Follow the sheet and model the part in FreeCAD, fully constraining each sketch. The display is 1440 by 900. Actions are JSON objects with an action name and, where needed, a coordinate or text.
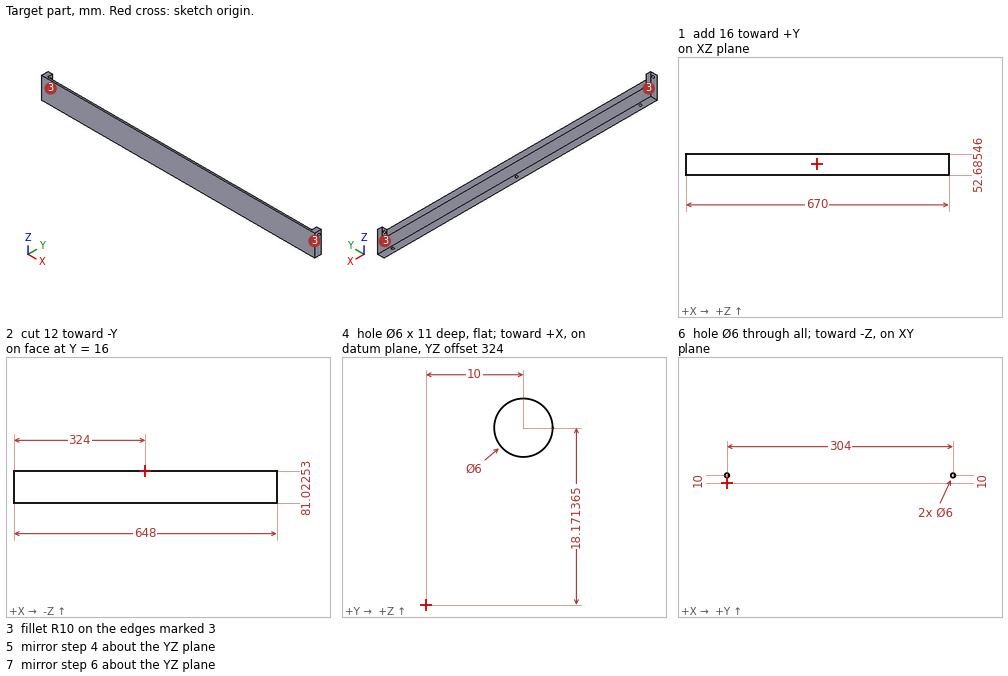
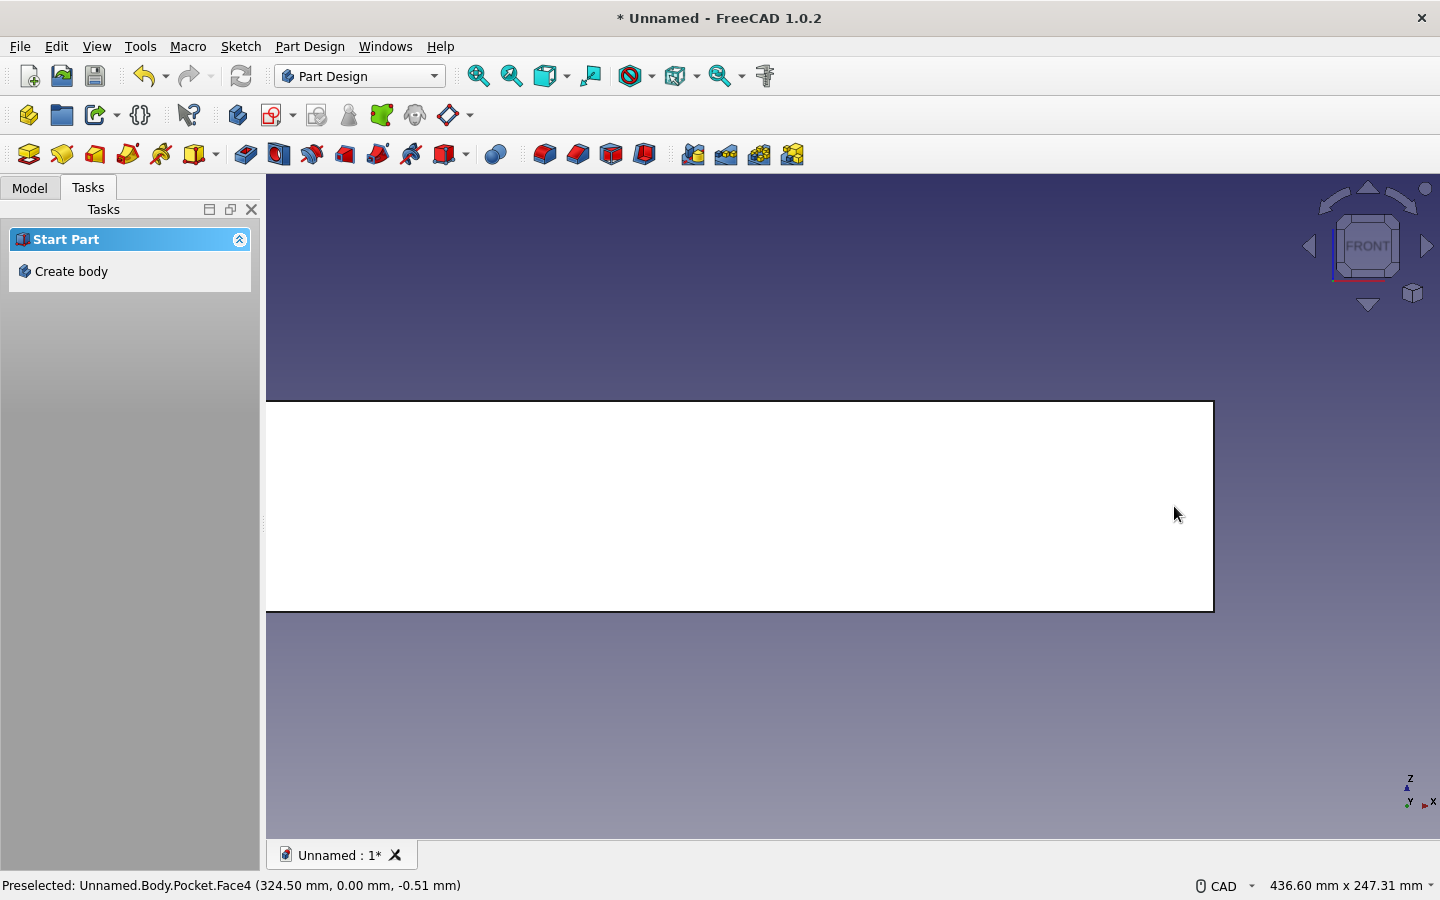
{"action": "left_click", "coordinate": [479, 76]}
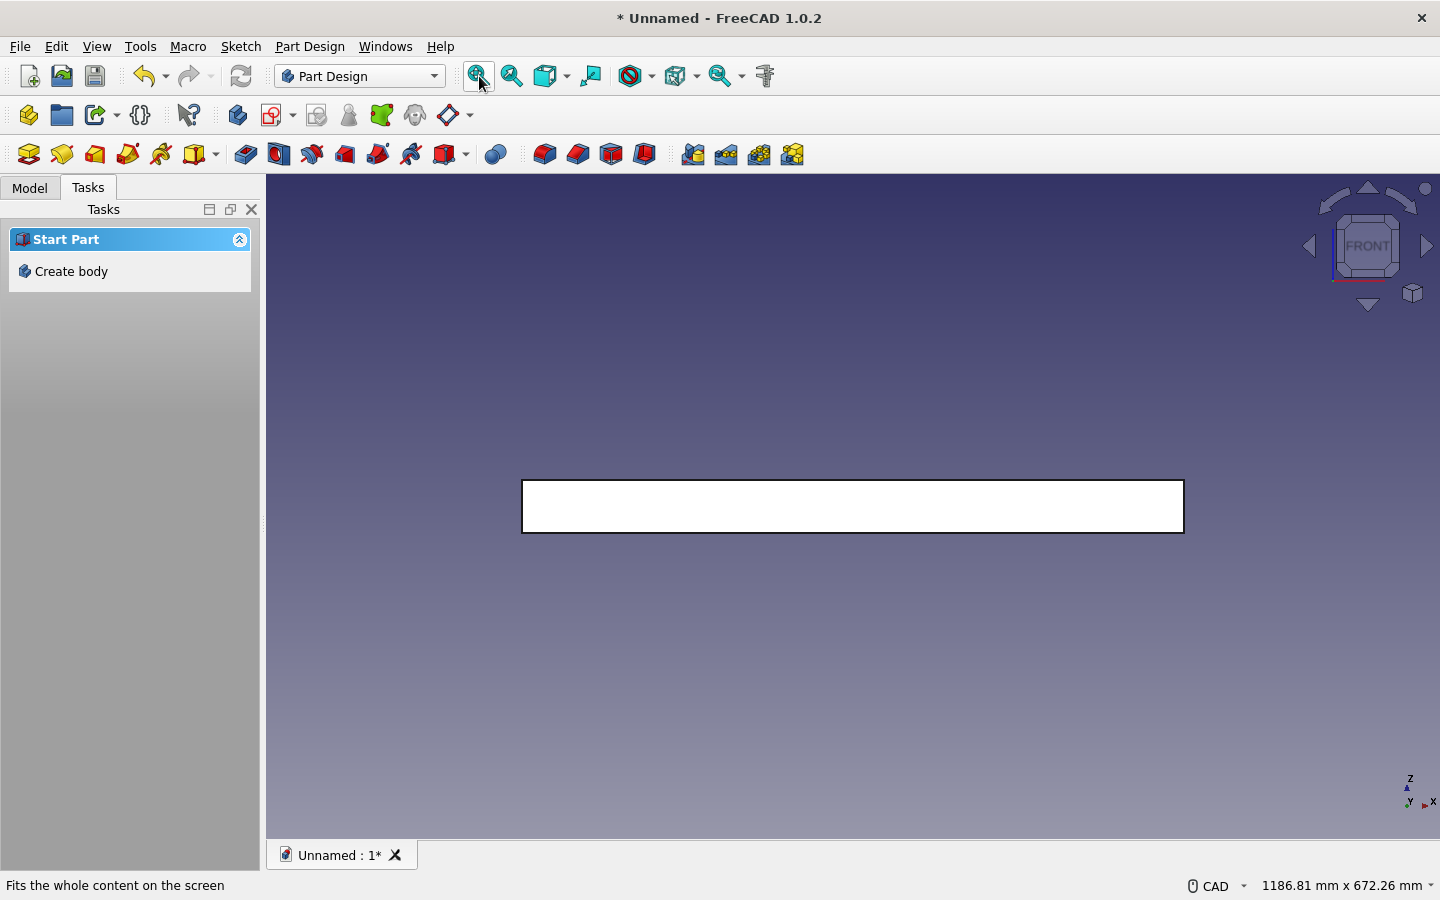
{"action": "key", "text": "3"}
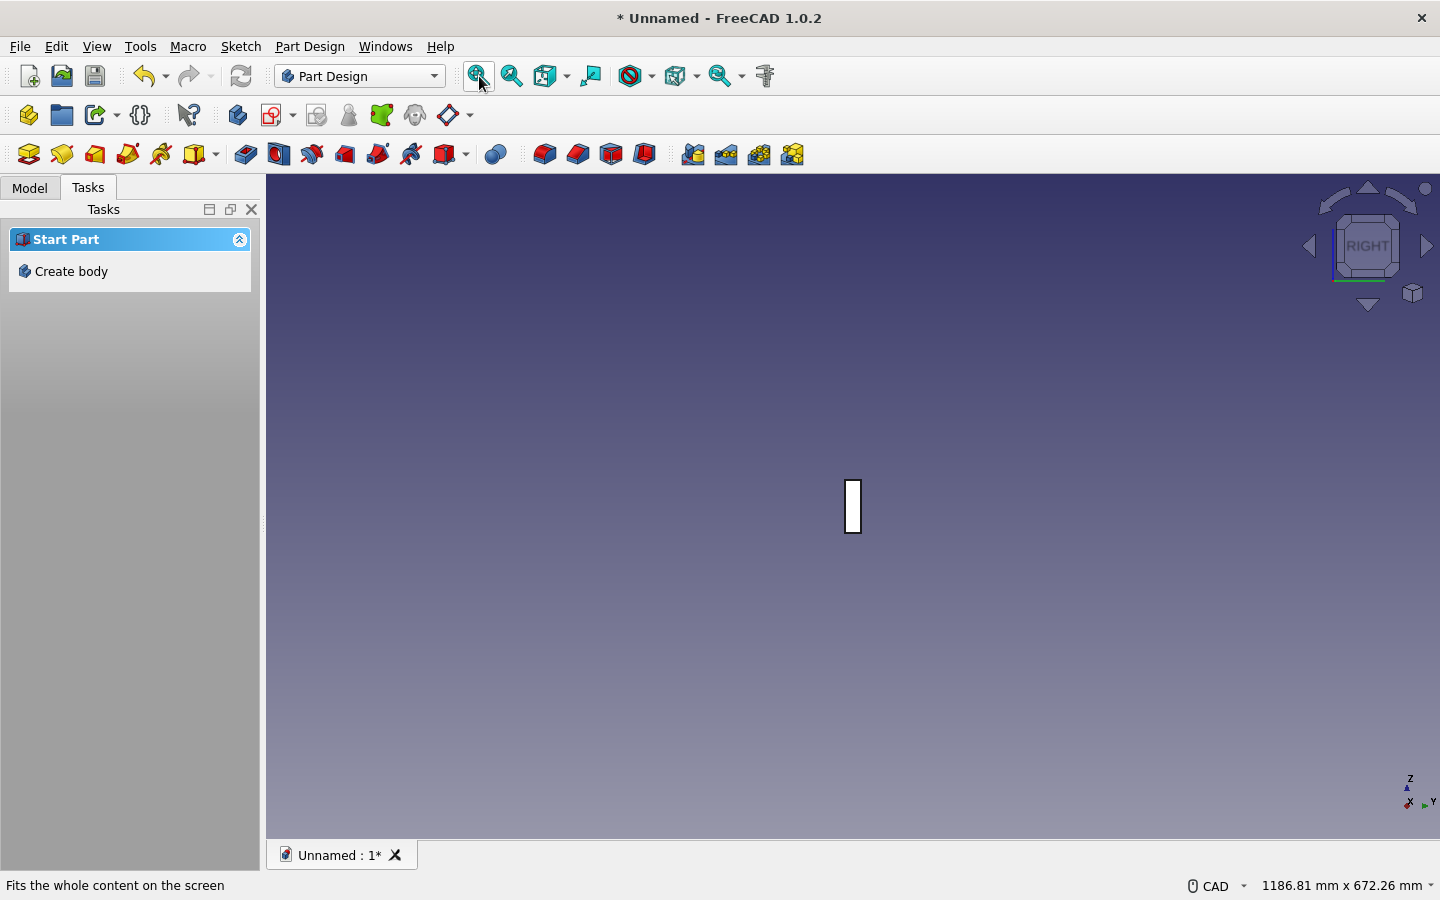
{"action": "left_click", "coordinate": [479, 76]}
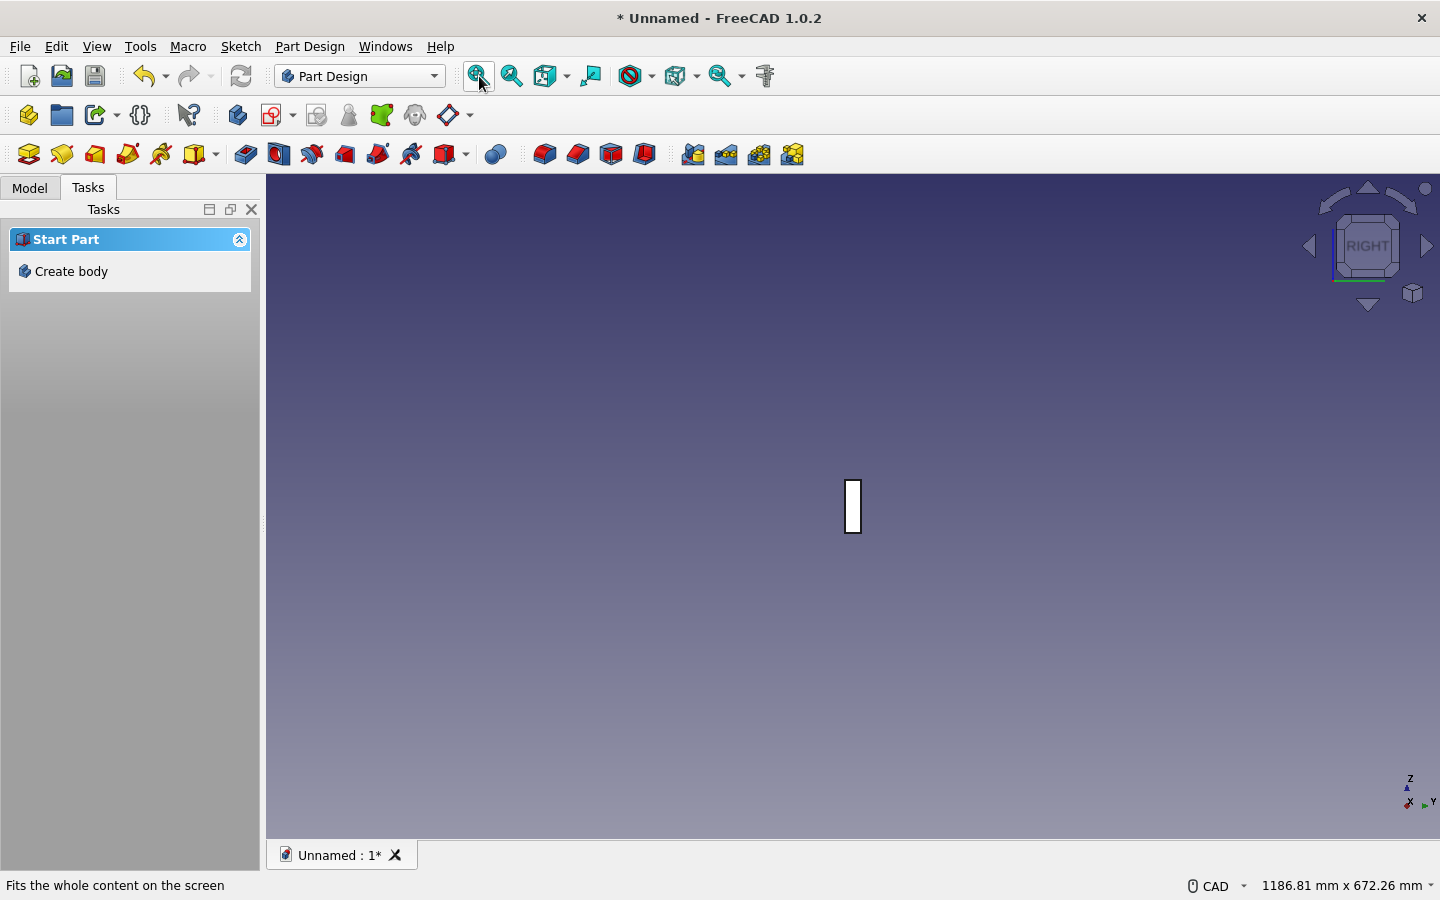
{"action": "scroll", "coordinate": [855, 505], "scroll_direction": "up", "scroll_amount": 7}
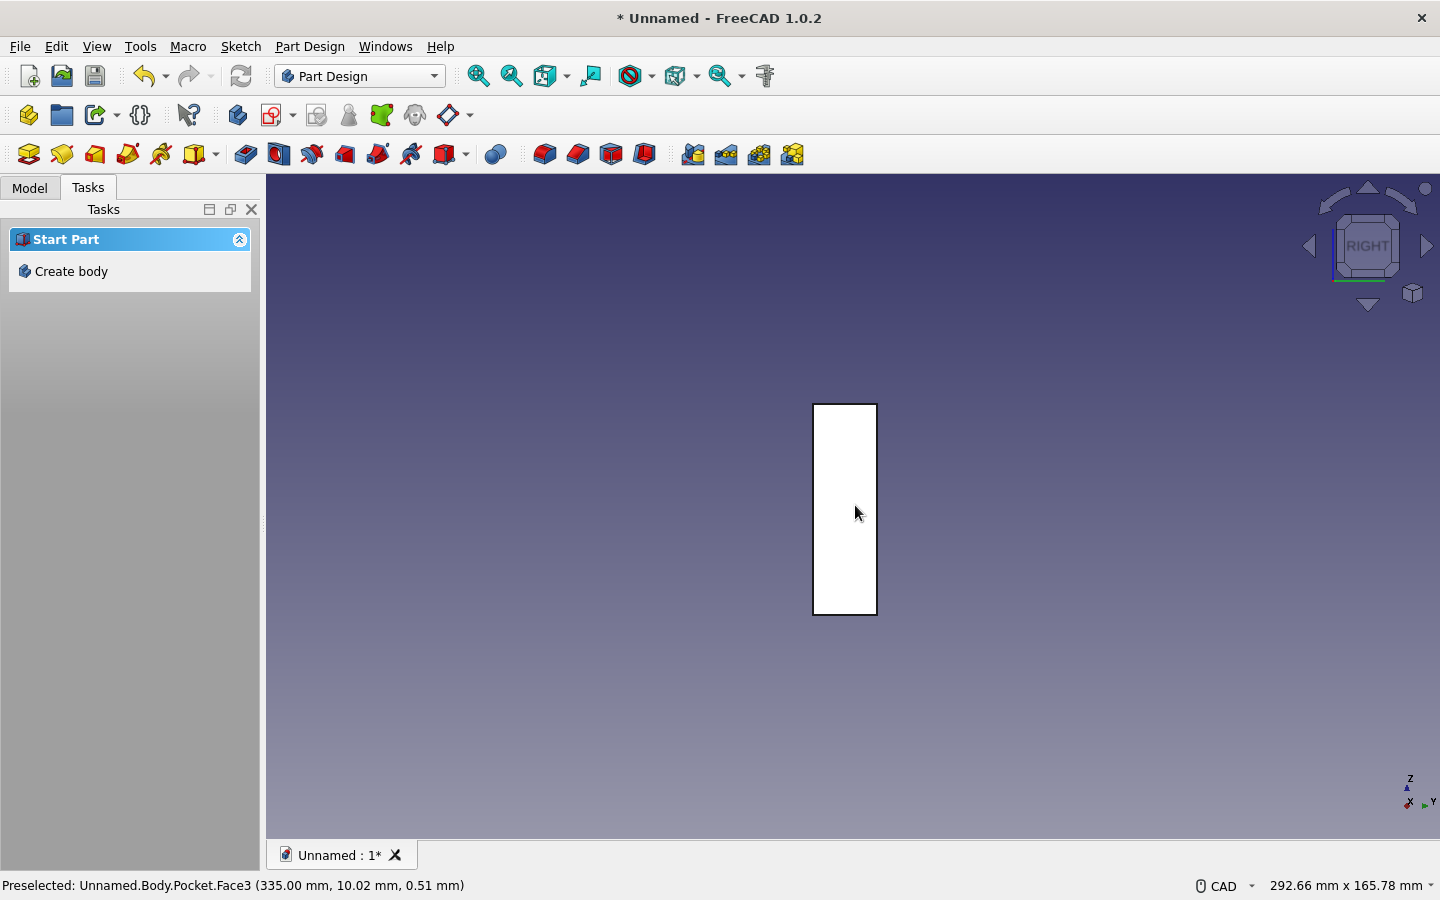
{"action": "left_click", "coordinate": [479, 76]}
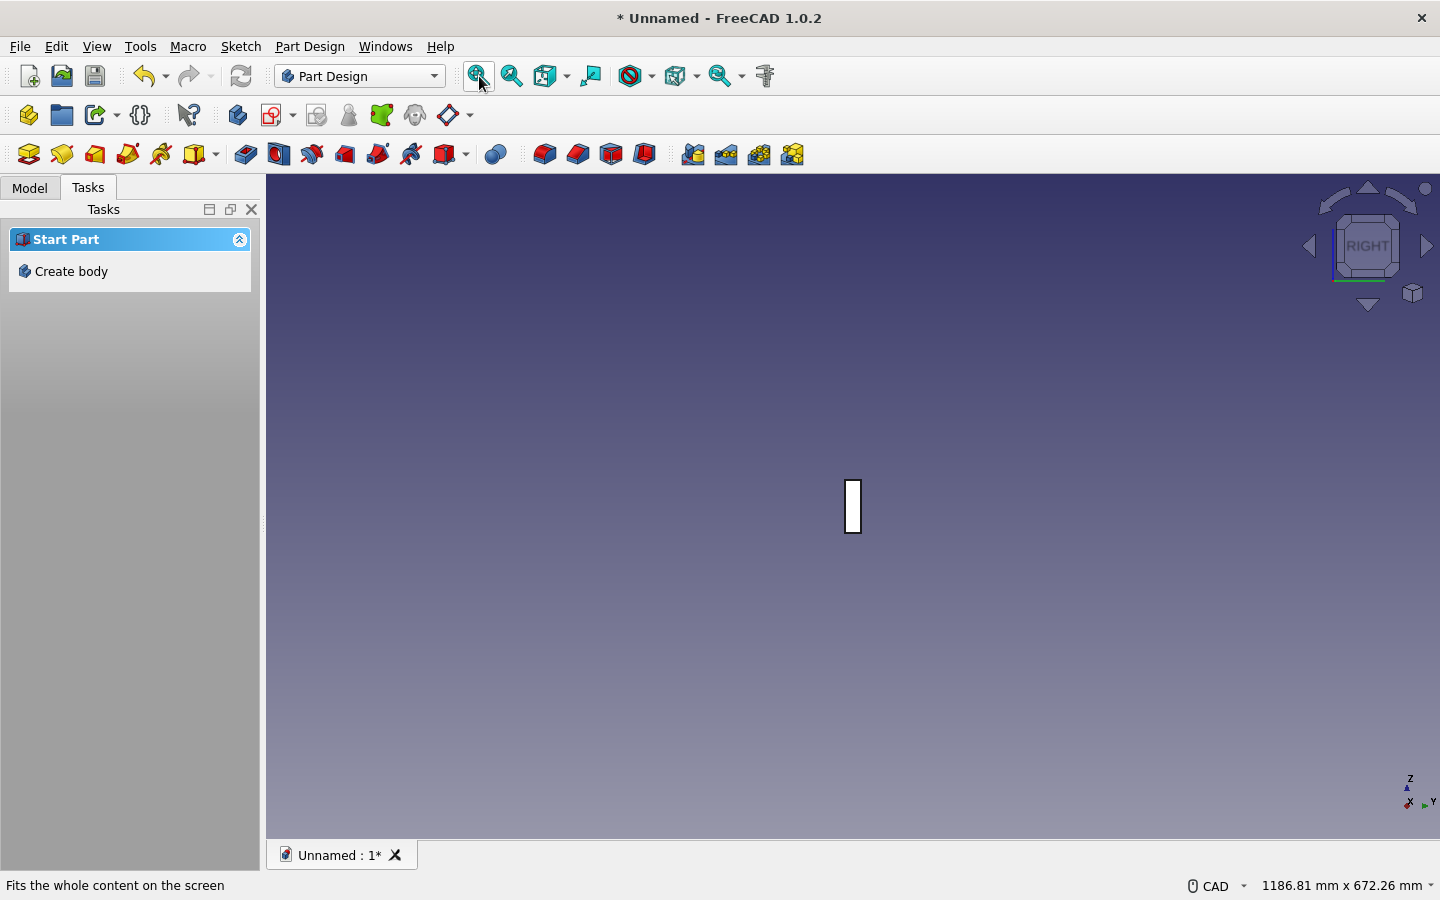
{"action": "key", "text": "5"}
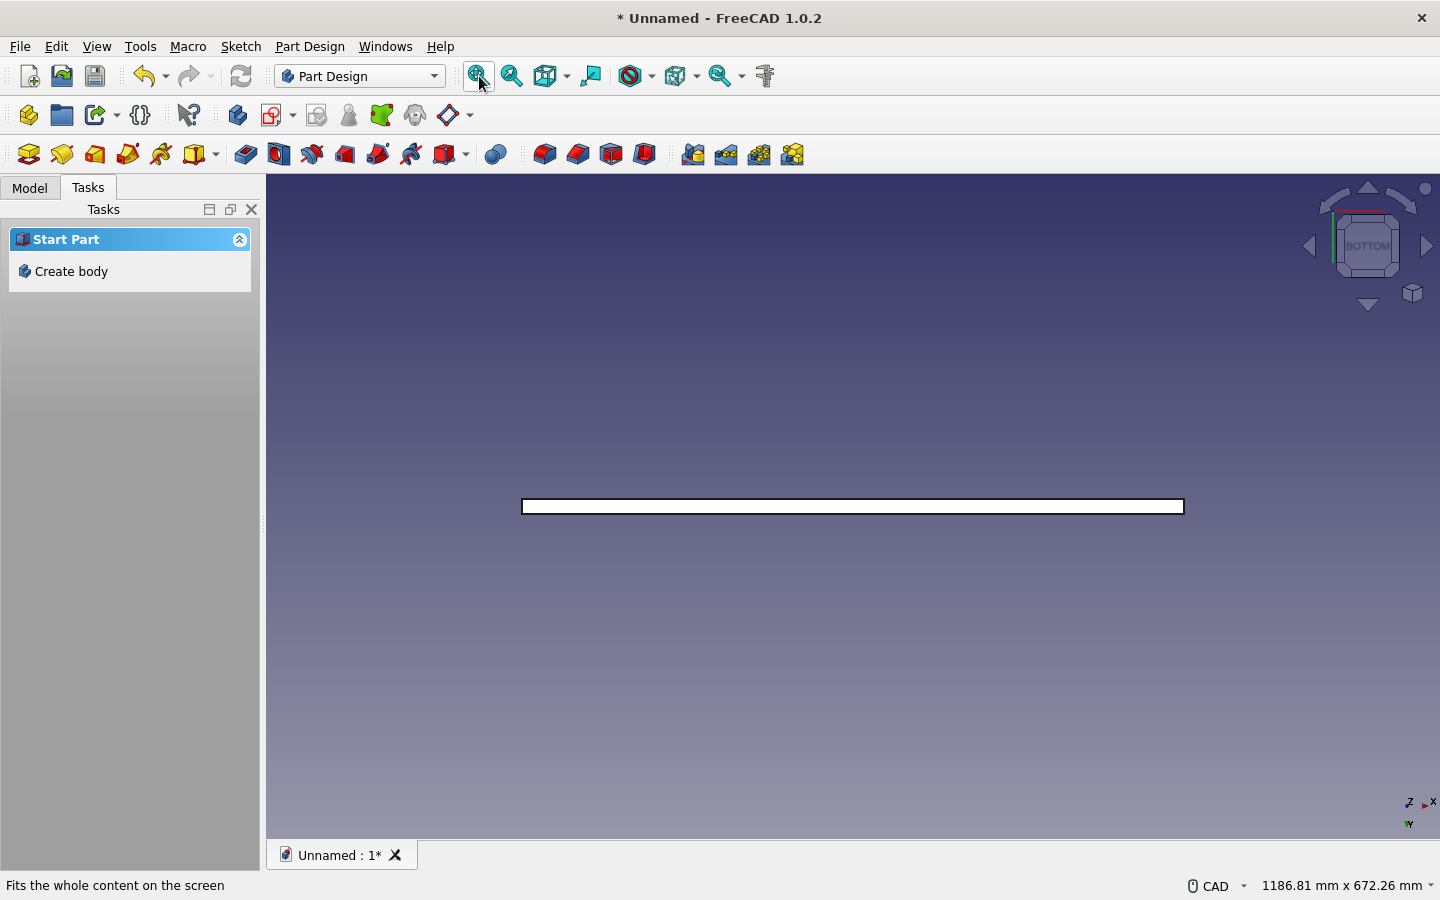
{"action": "scroll", "coordinate": [1174, 507], "scroll_direction": "up", "scroll_amount": 7}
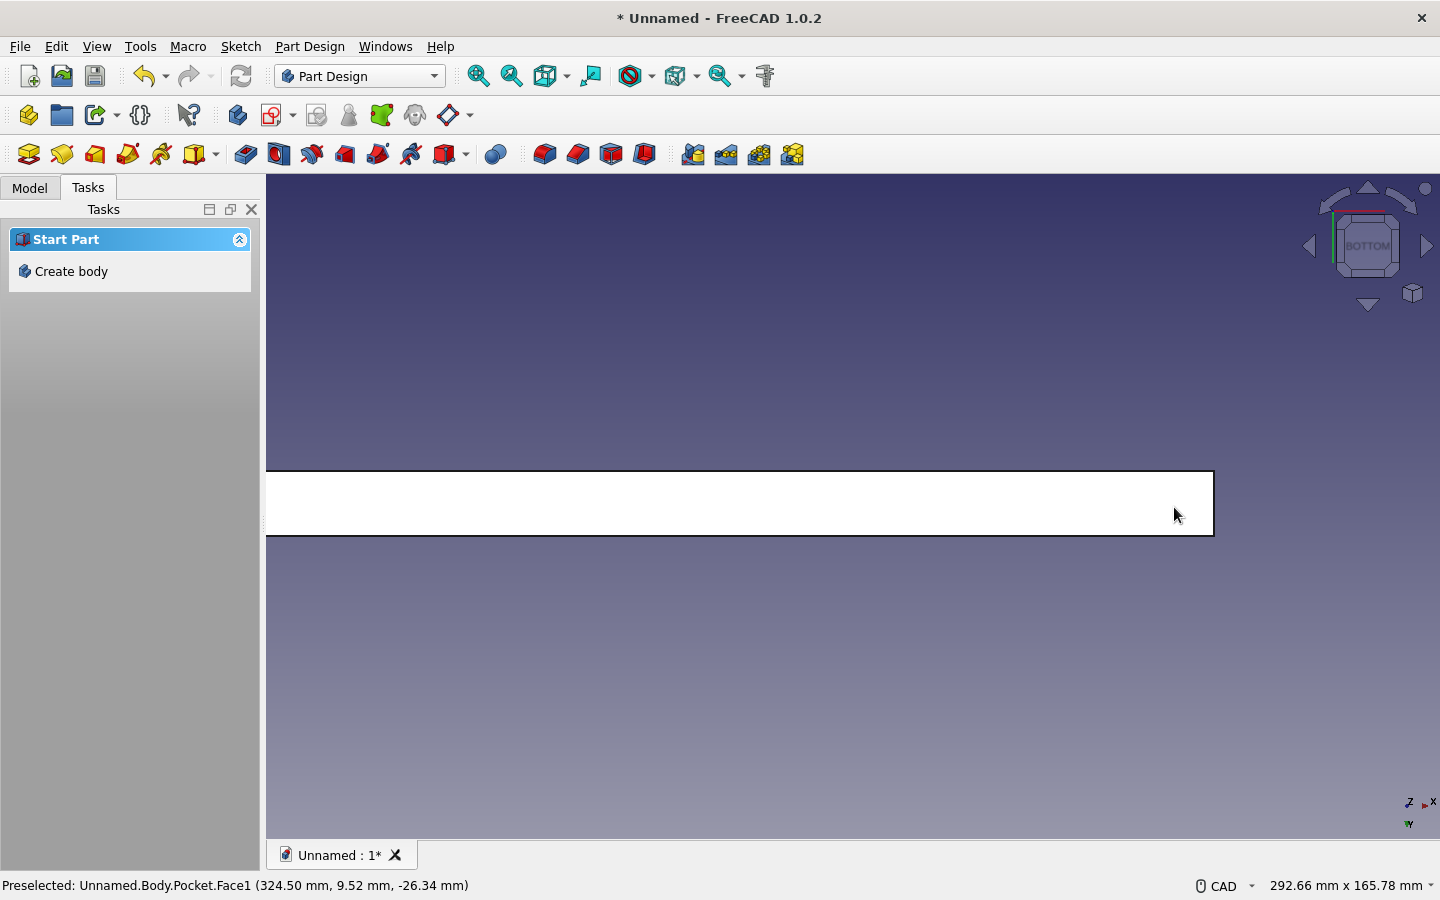
{"action": "left_click", "coordinate": [479, 76]}